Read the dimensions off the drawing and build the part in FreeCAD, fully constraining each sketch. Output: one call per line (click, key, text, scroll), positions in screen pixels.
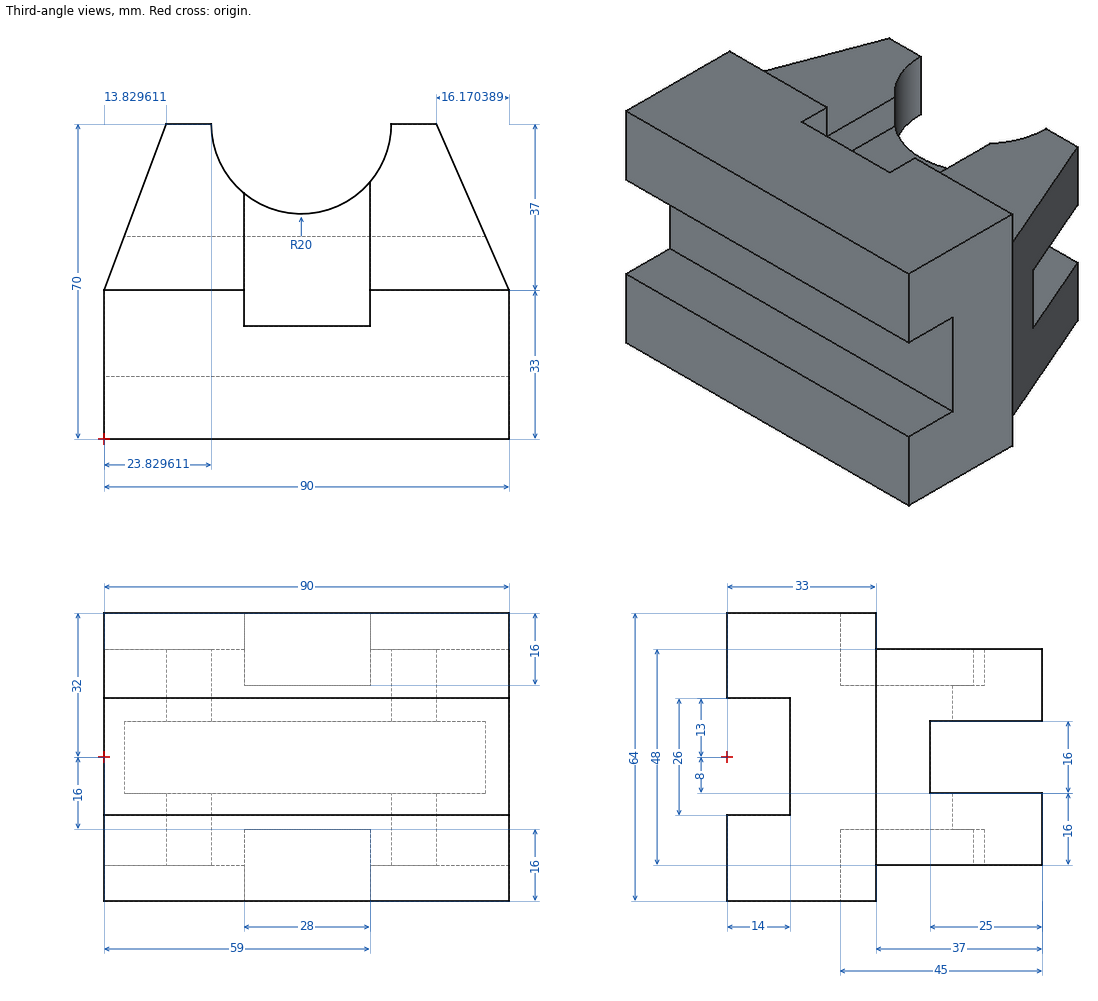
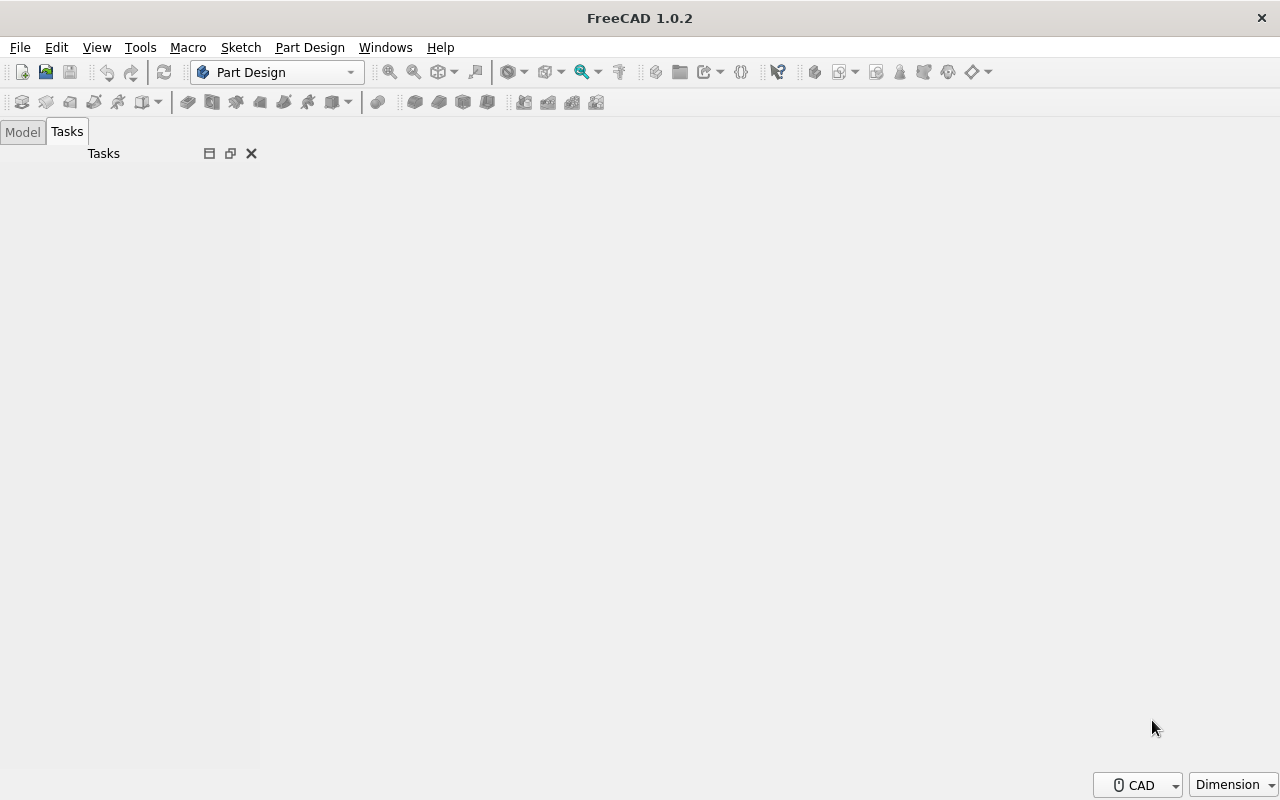
click(22, 72)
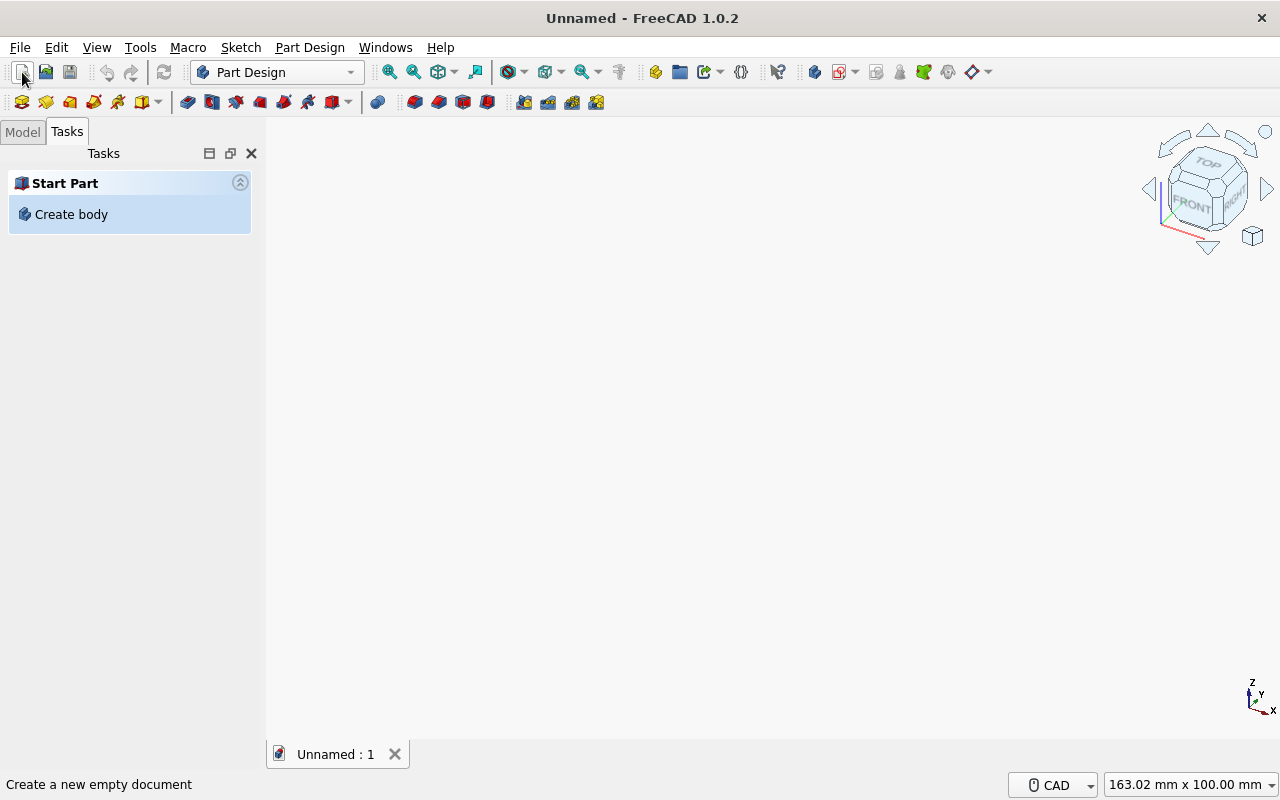
click(840, 72)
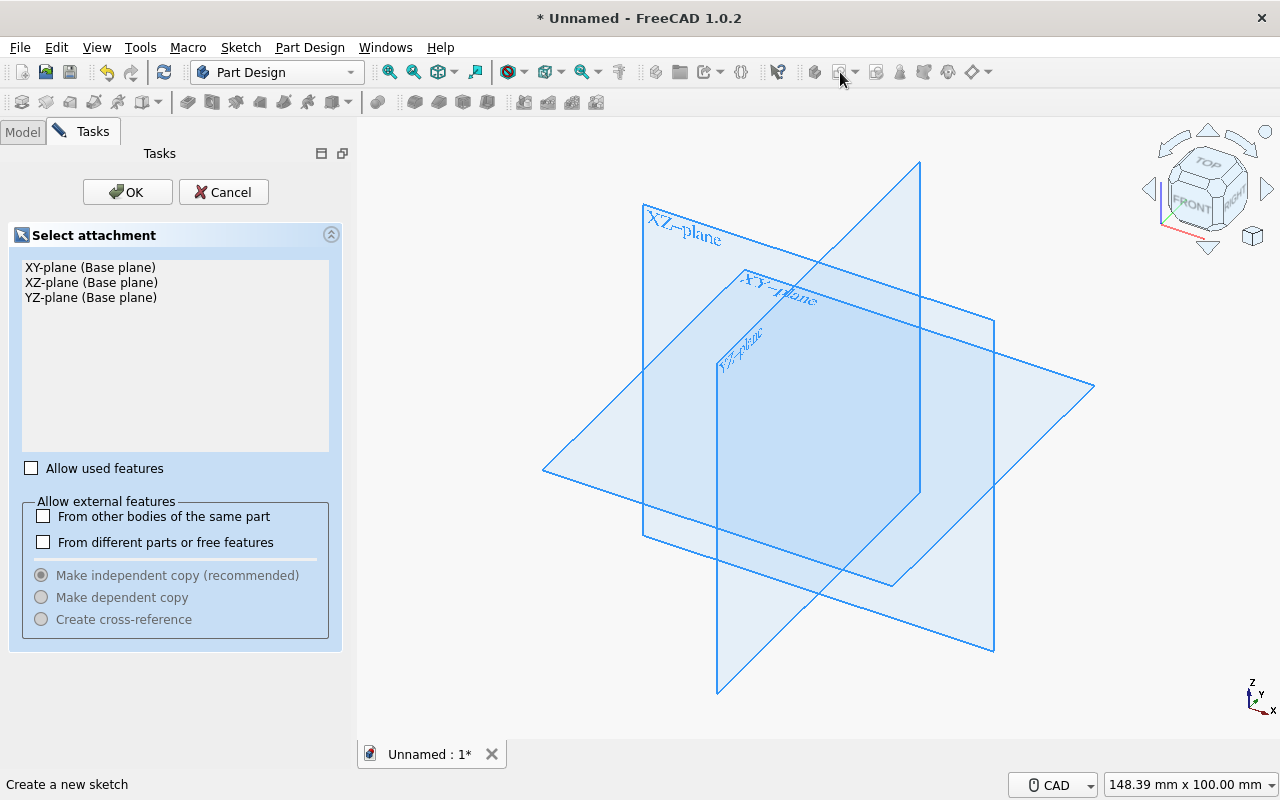
click(82, 268)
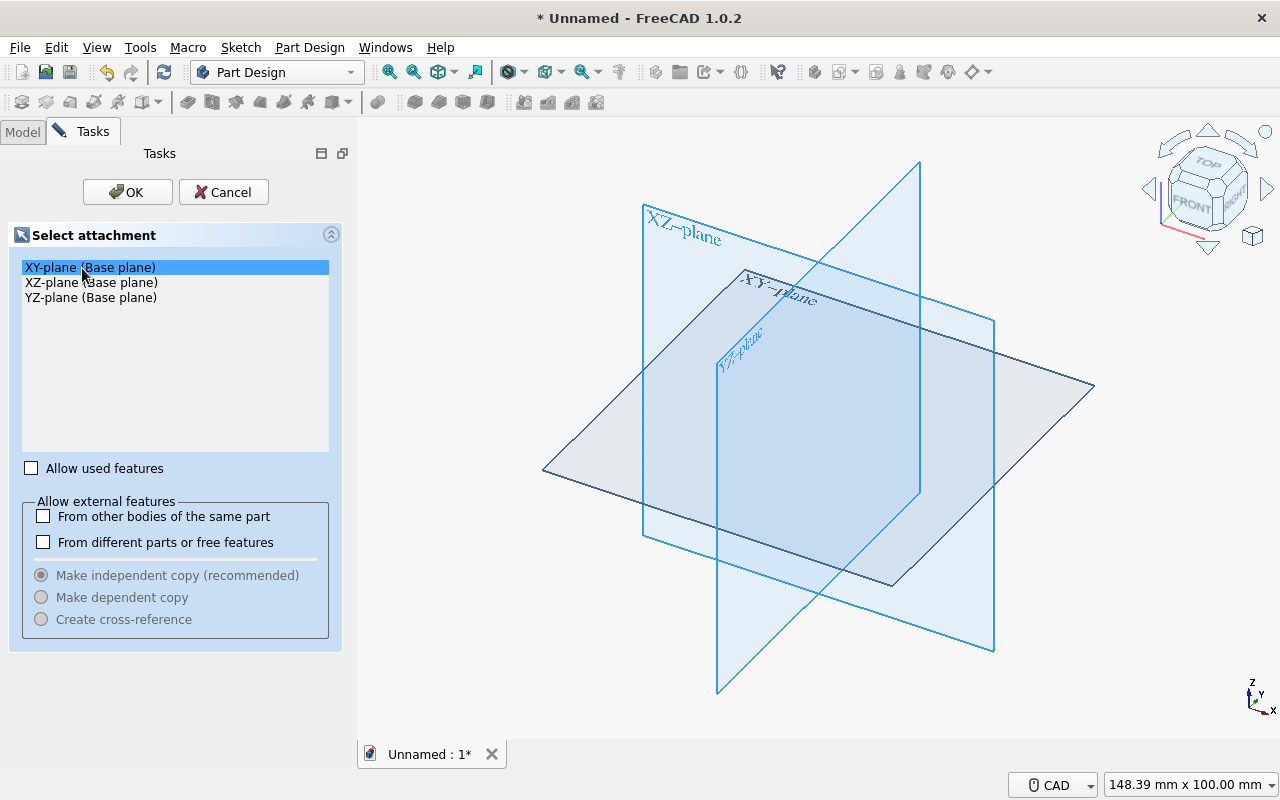
click(128, 192)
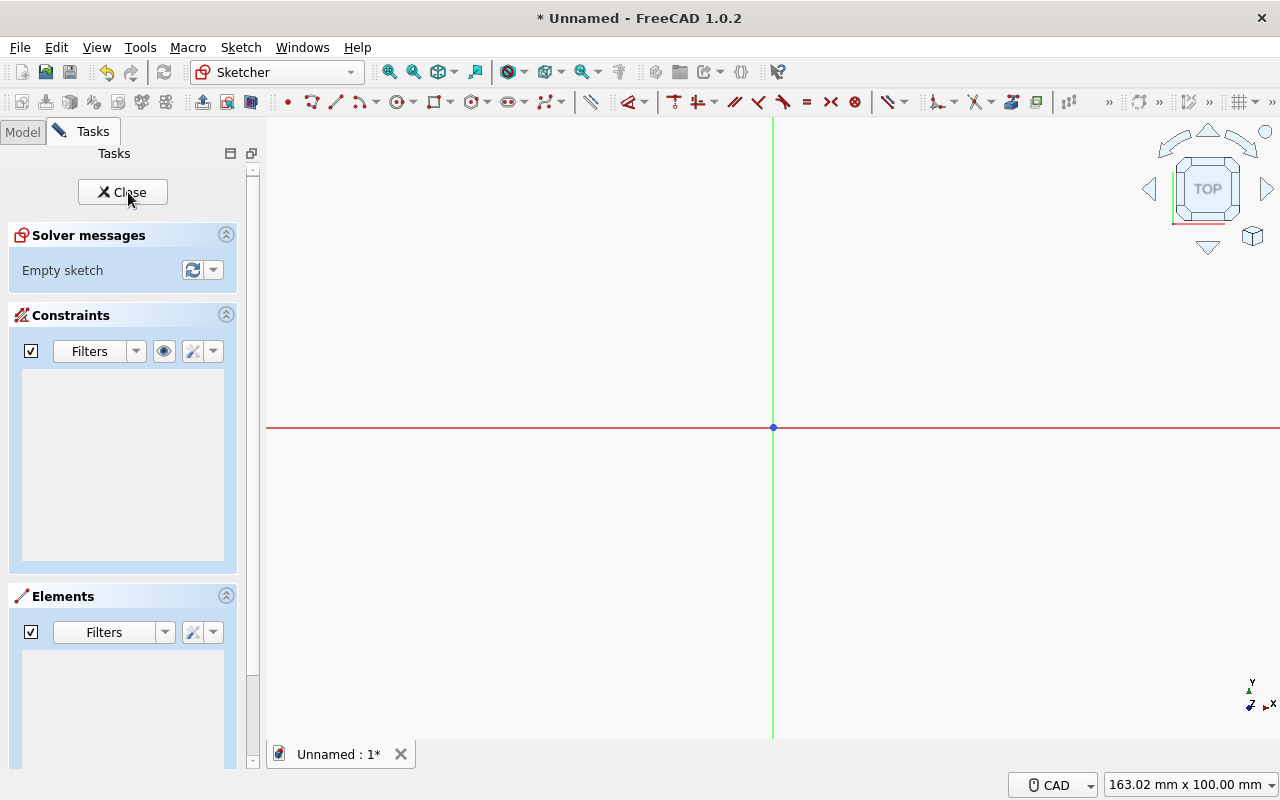
scroll(294, 637, down, 2)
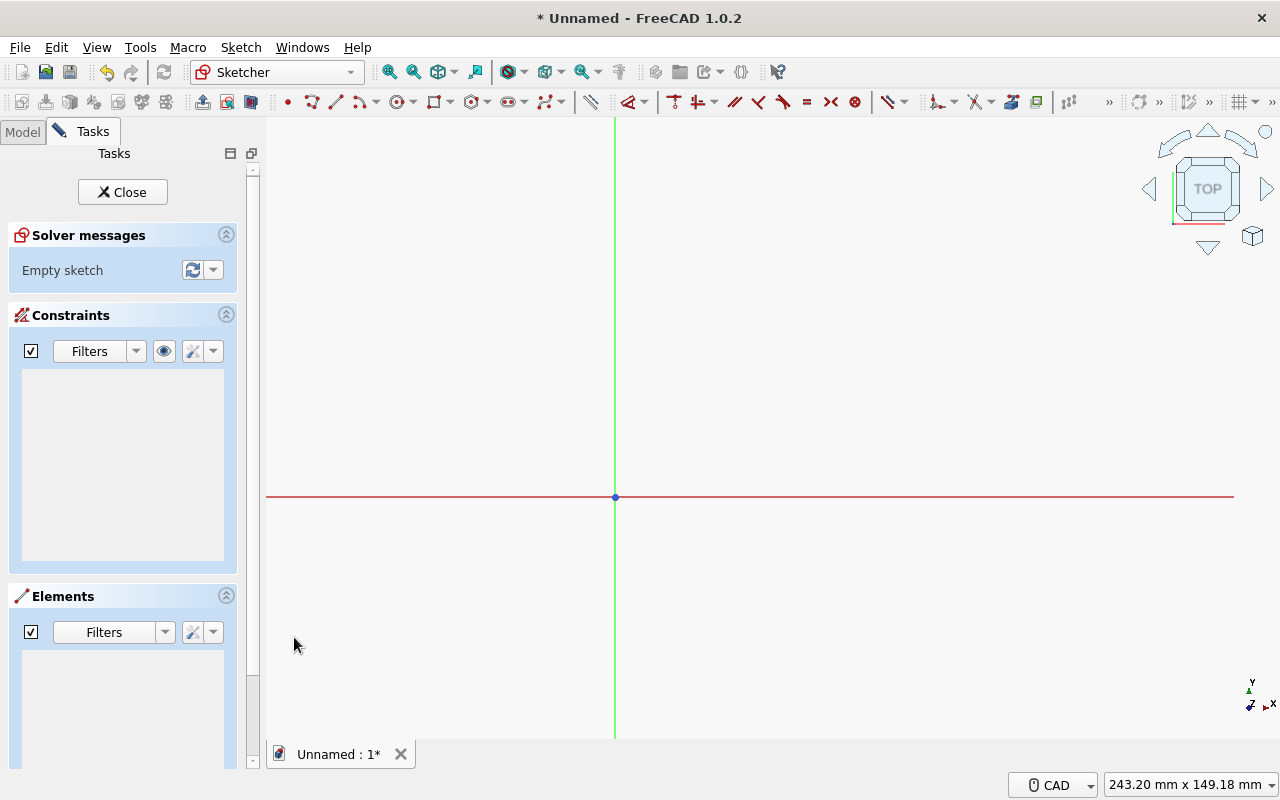
scroll(1002, 429, up, 2)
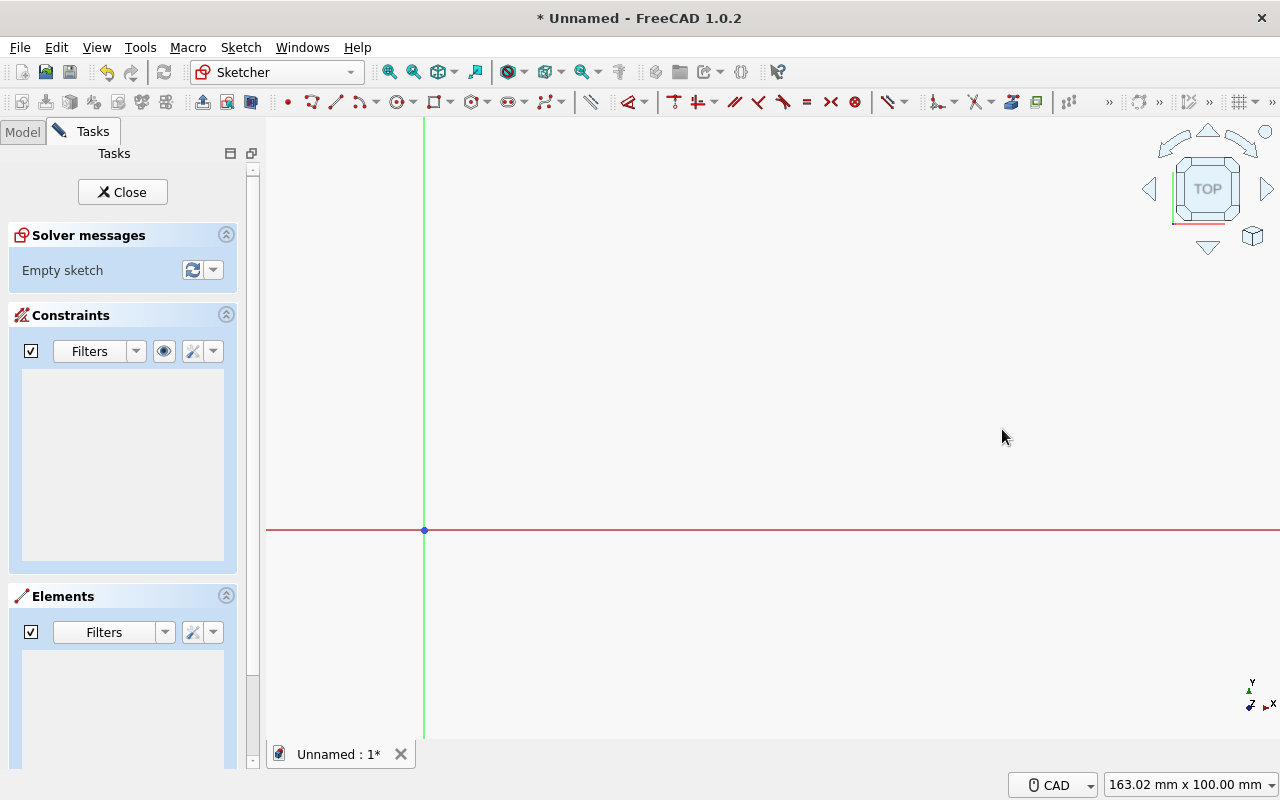
key(g)
key(r)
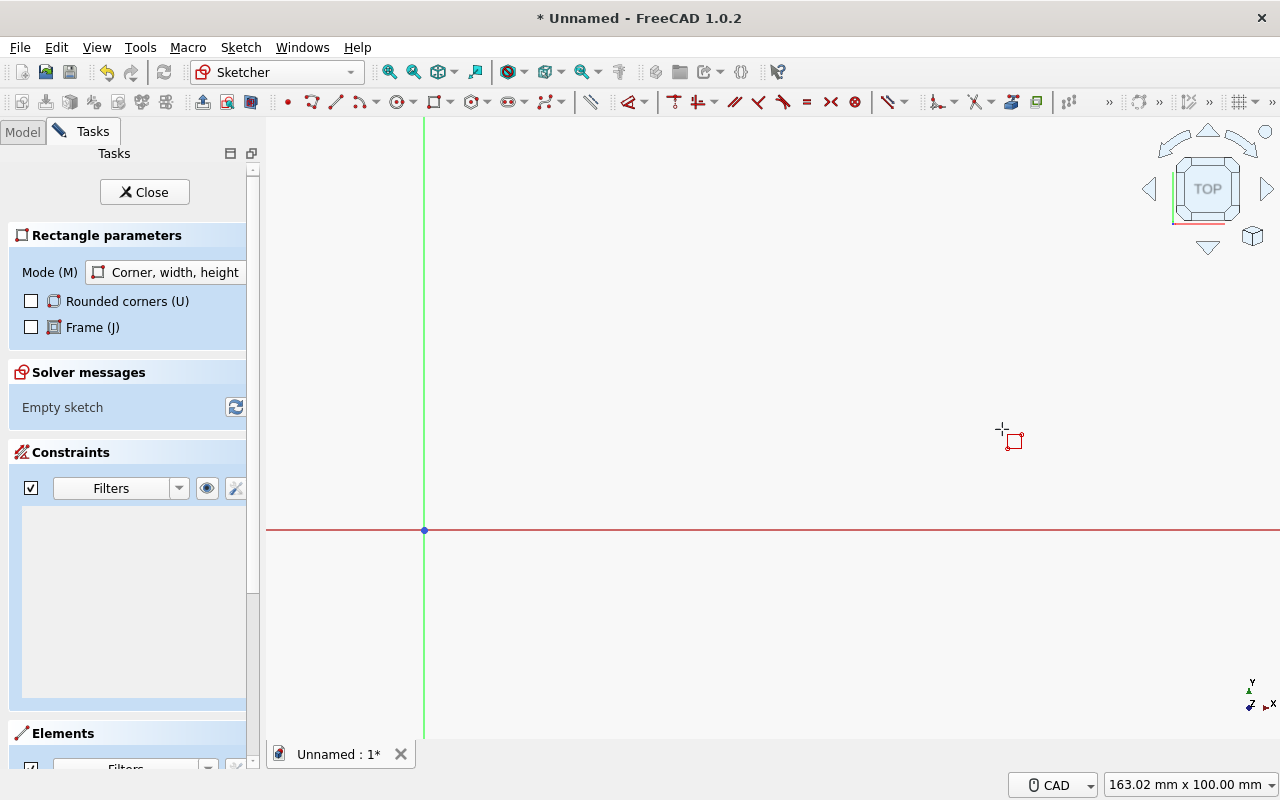
click(424, 530)
click(984, 325)
key(Escape)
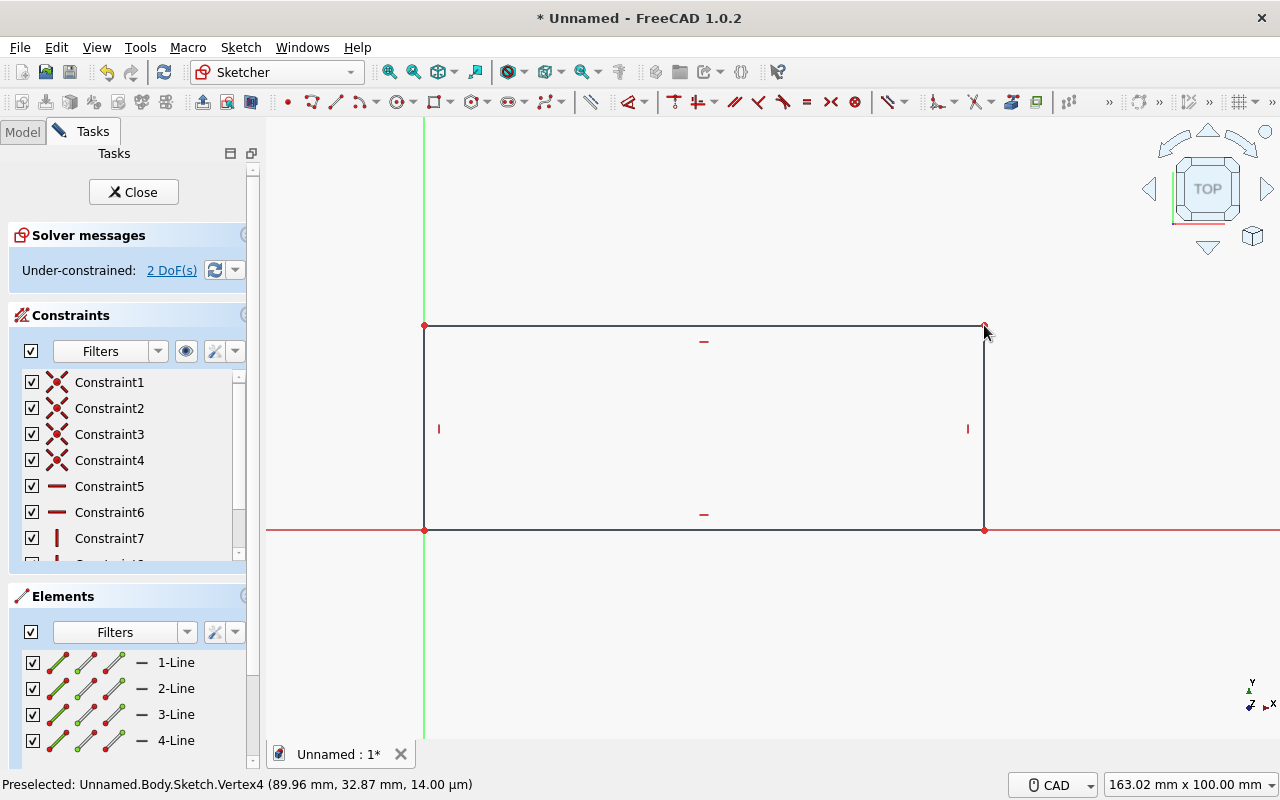
click(628, 102)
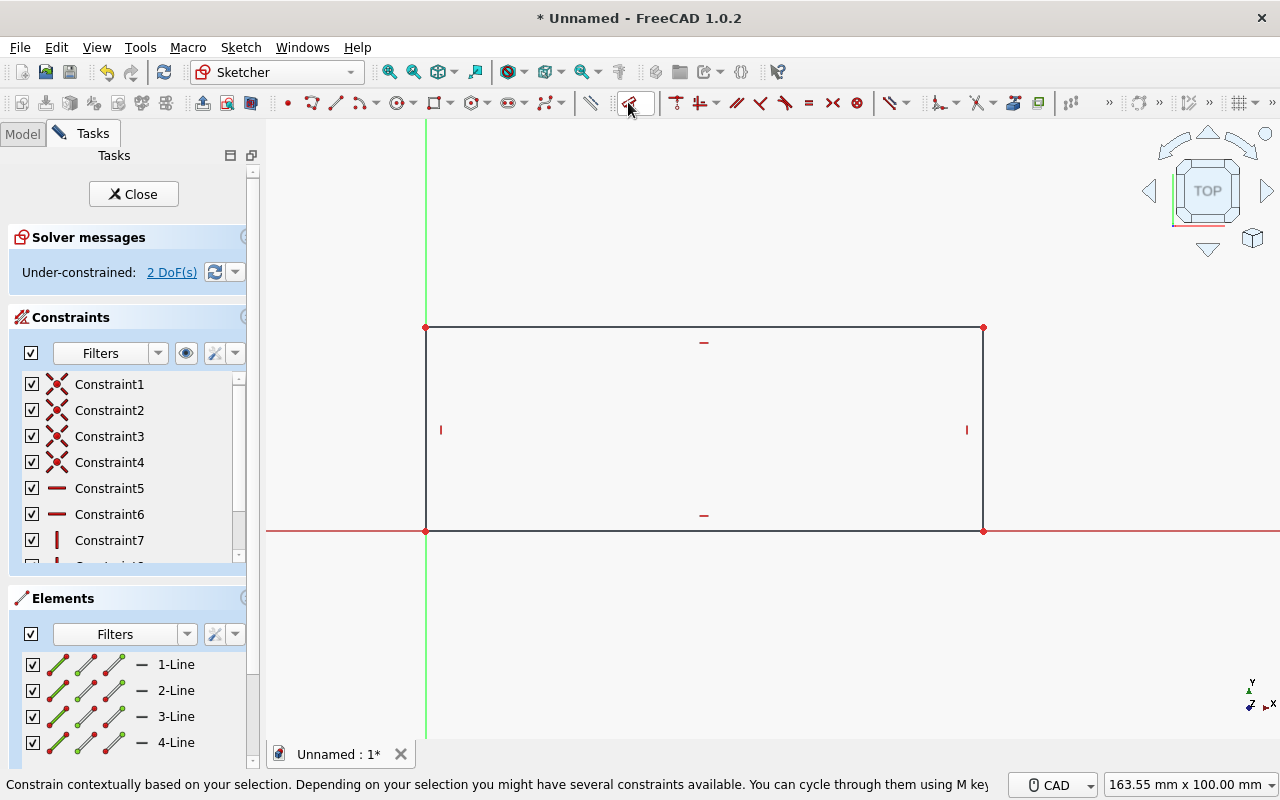
click(593, 531)
click(704, 565)